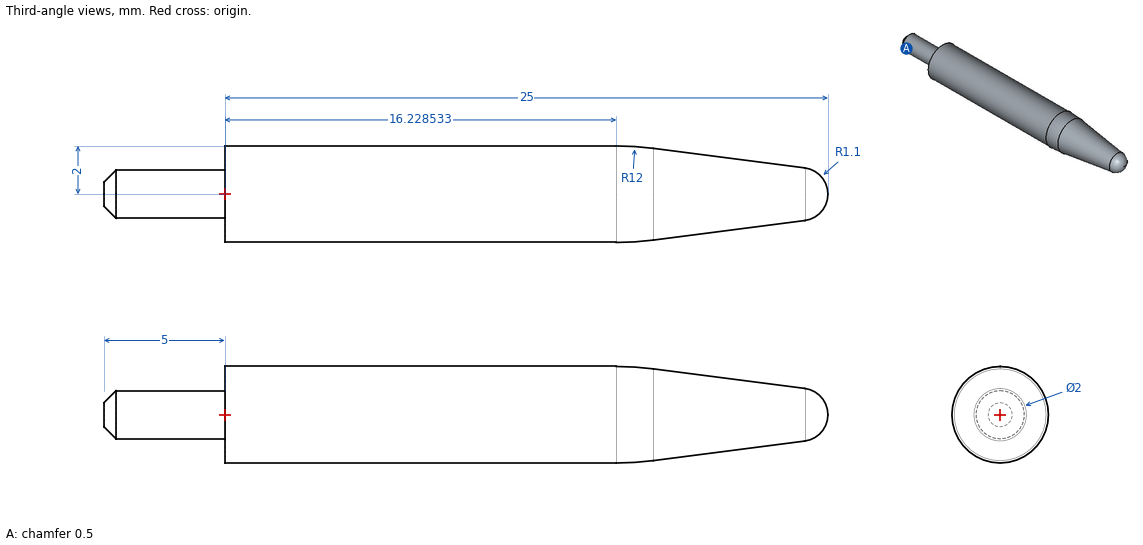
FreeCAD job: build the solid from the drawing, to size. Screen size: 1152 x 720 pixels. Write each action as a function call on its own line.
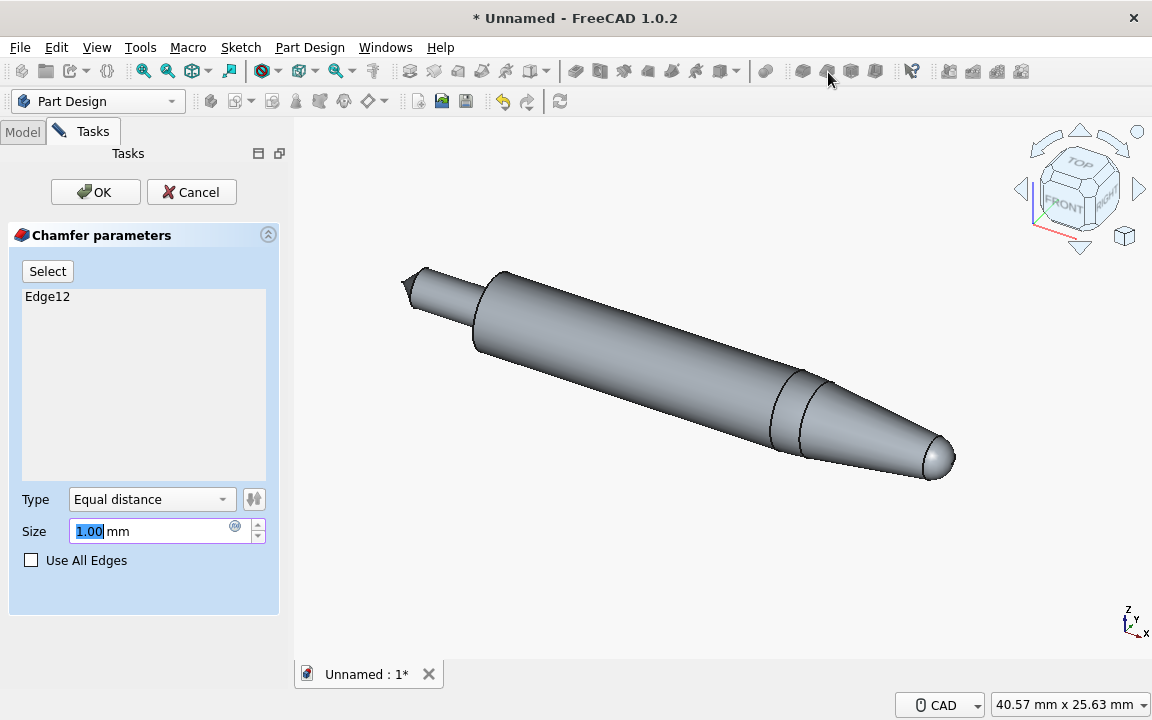
text(0.5)
key(Tab)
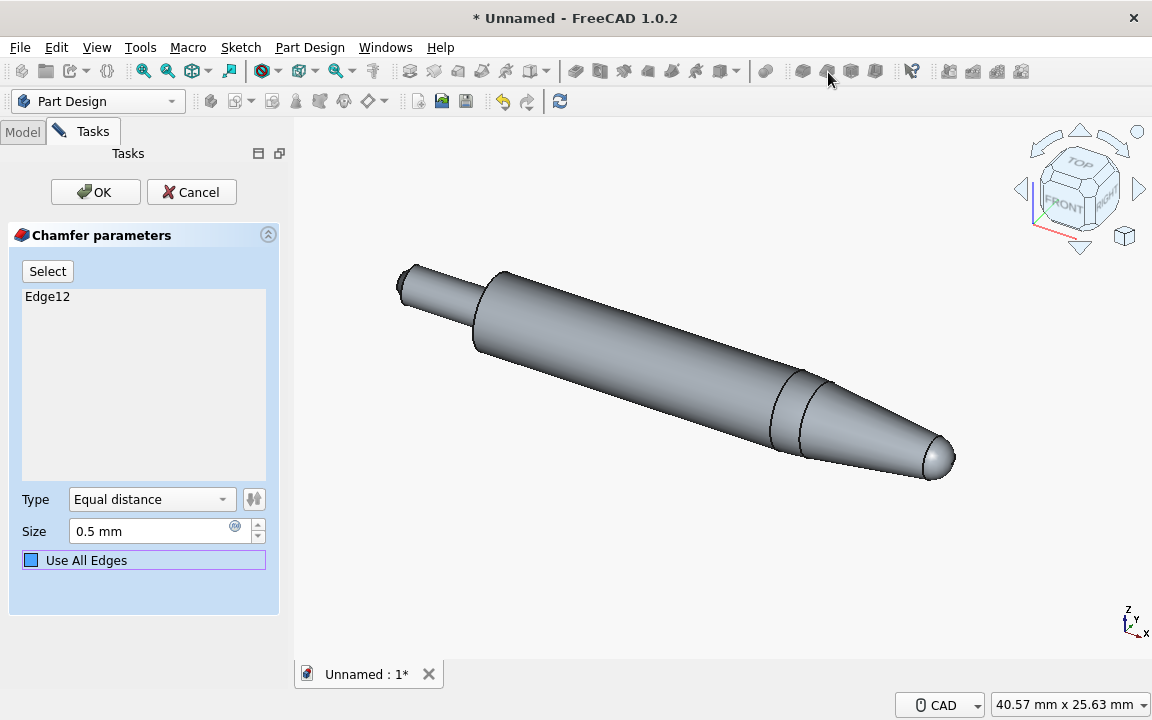
click(96, 192)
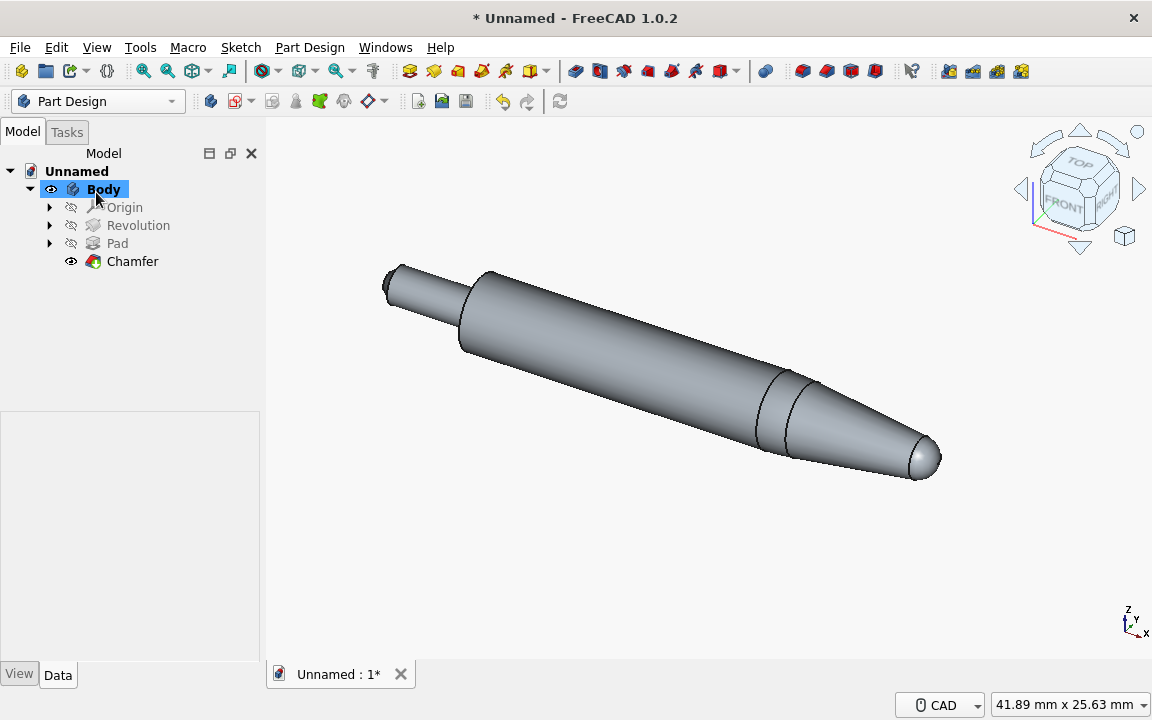
key(0)